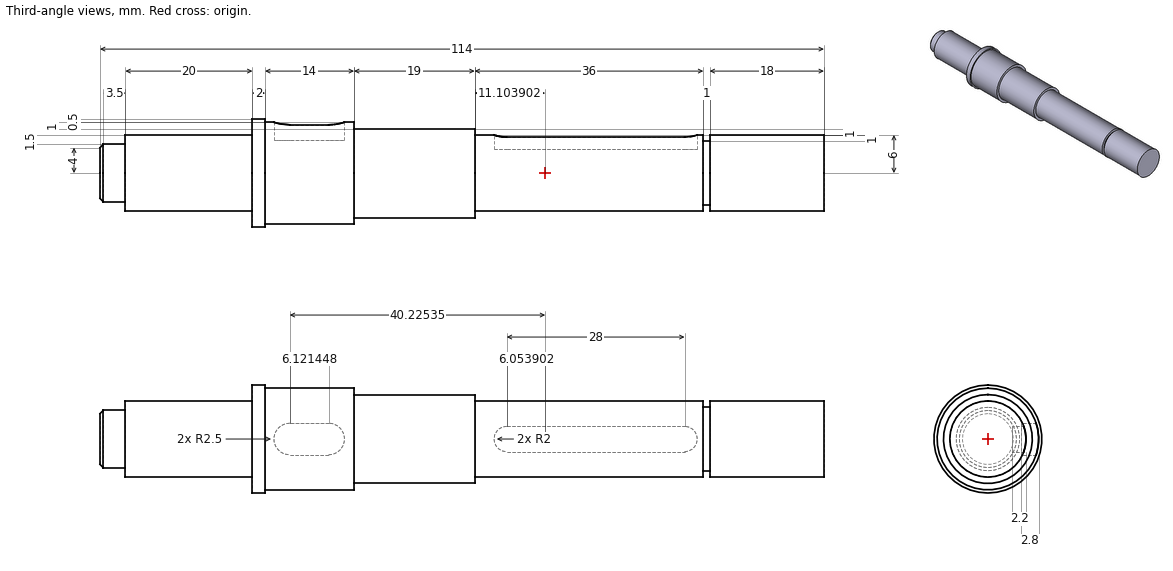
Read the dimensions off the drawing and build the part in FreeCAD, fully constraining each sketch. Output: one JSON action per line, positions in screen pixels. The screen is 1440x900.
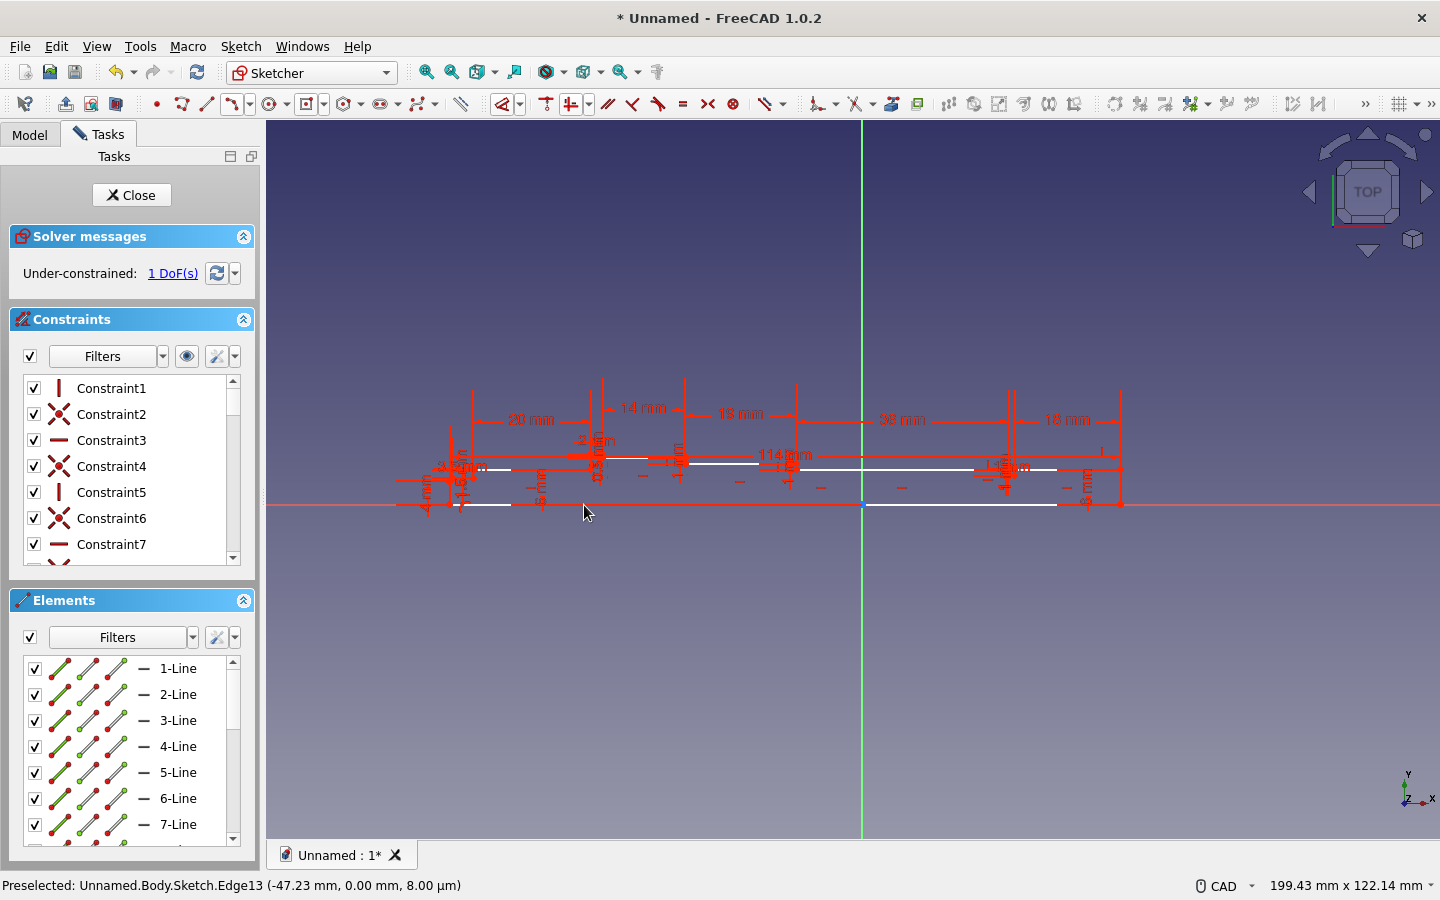
{"action": "scroll", "coordinate": [797, 470], "scroll_direction": "up", "scroll_amount": 4}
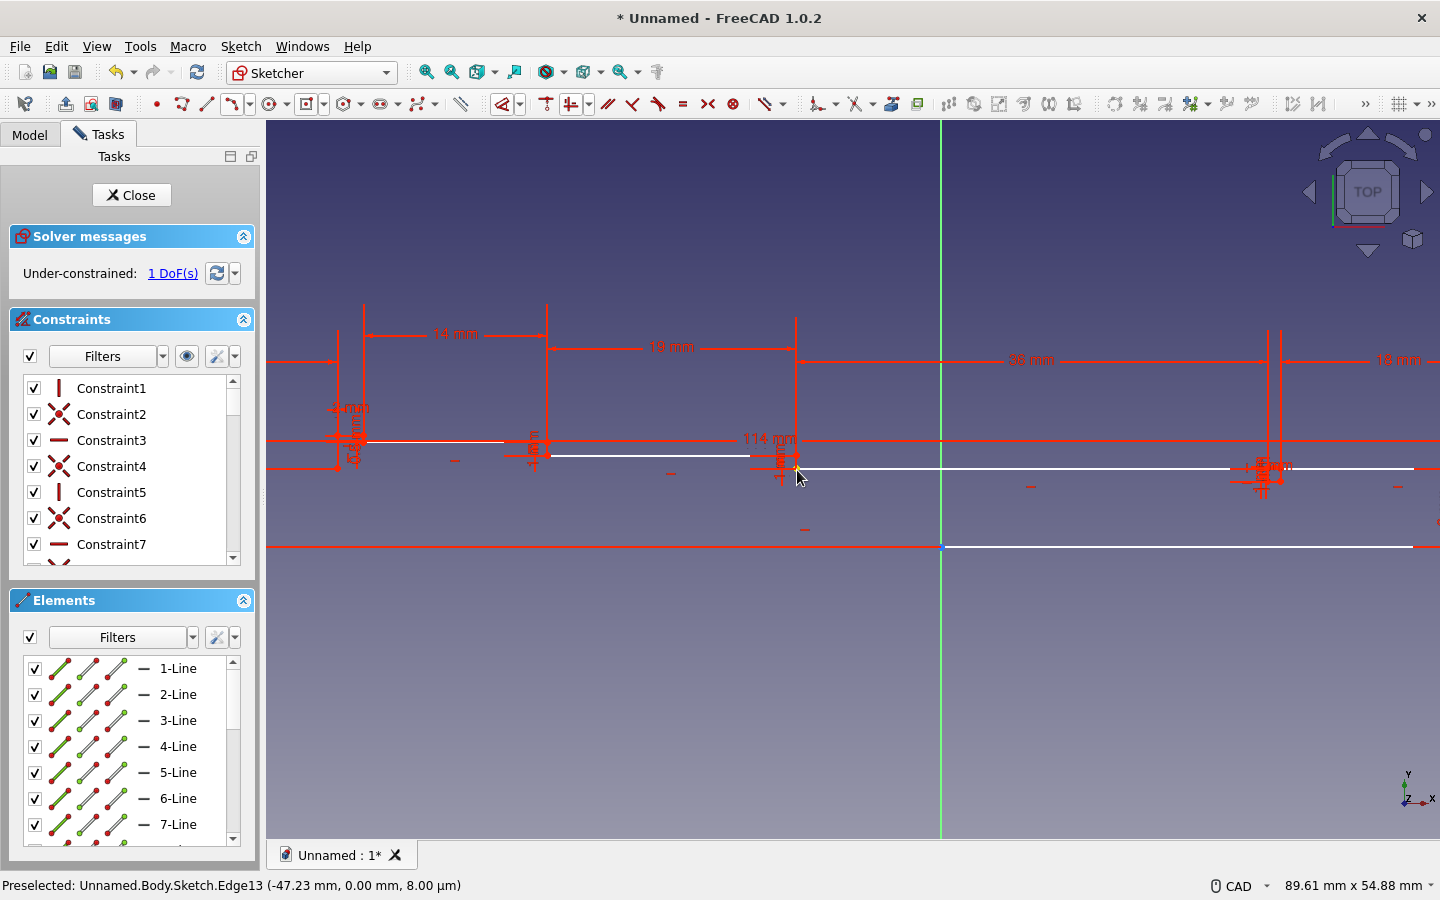
{"action": "left_click", "coordinate": [796, 469]}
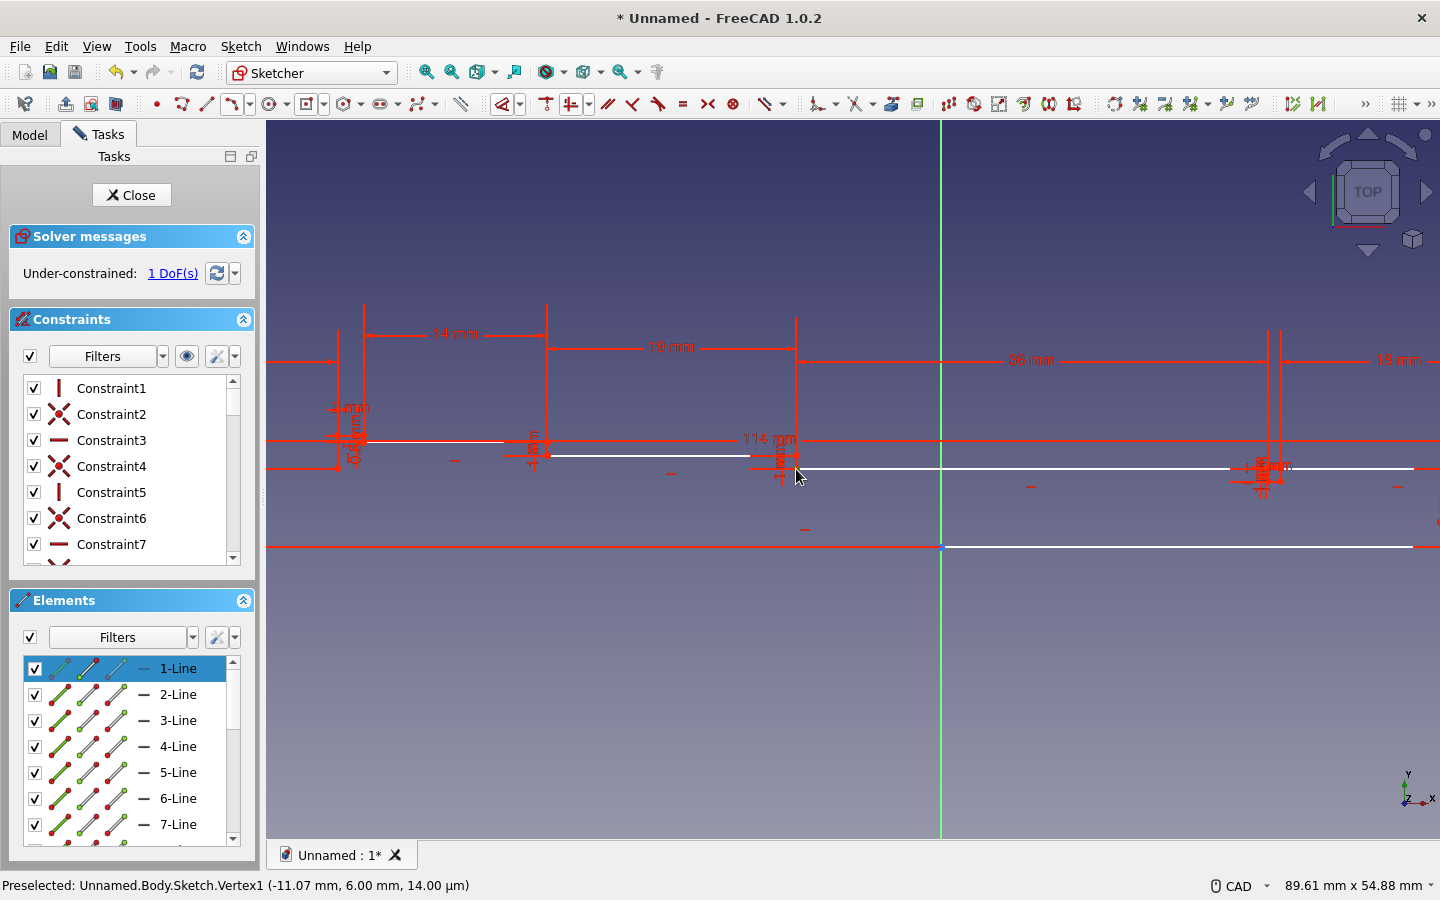
{"action": "key", "text": "l"}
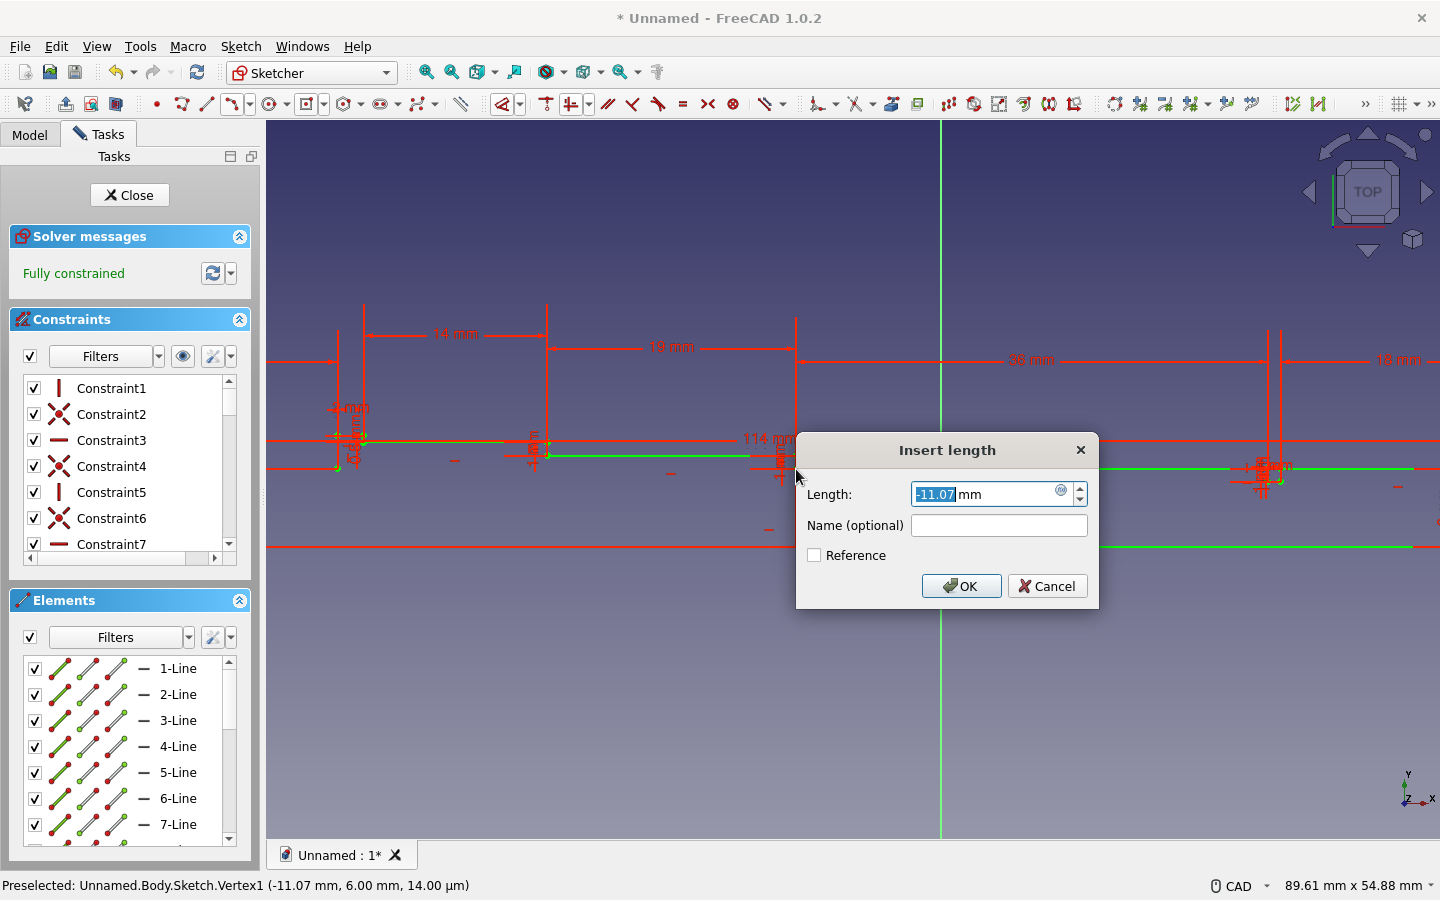
{"action": "type", "text": "-11.103902"}
{"action": "key", "text": "Return"}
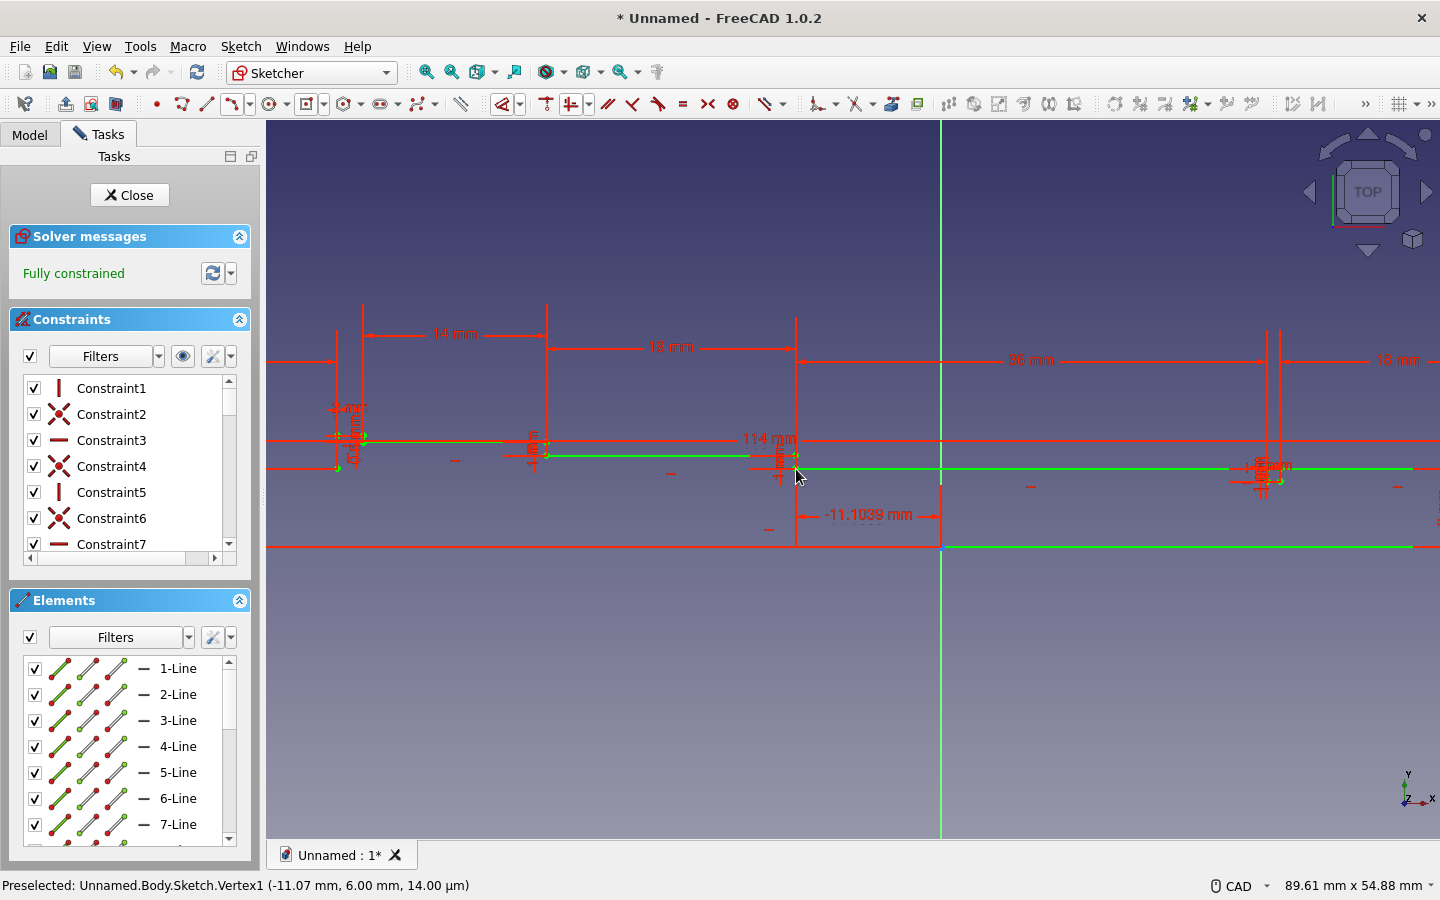
{"action": "left_click", "coordinate": [130, 195]}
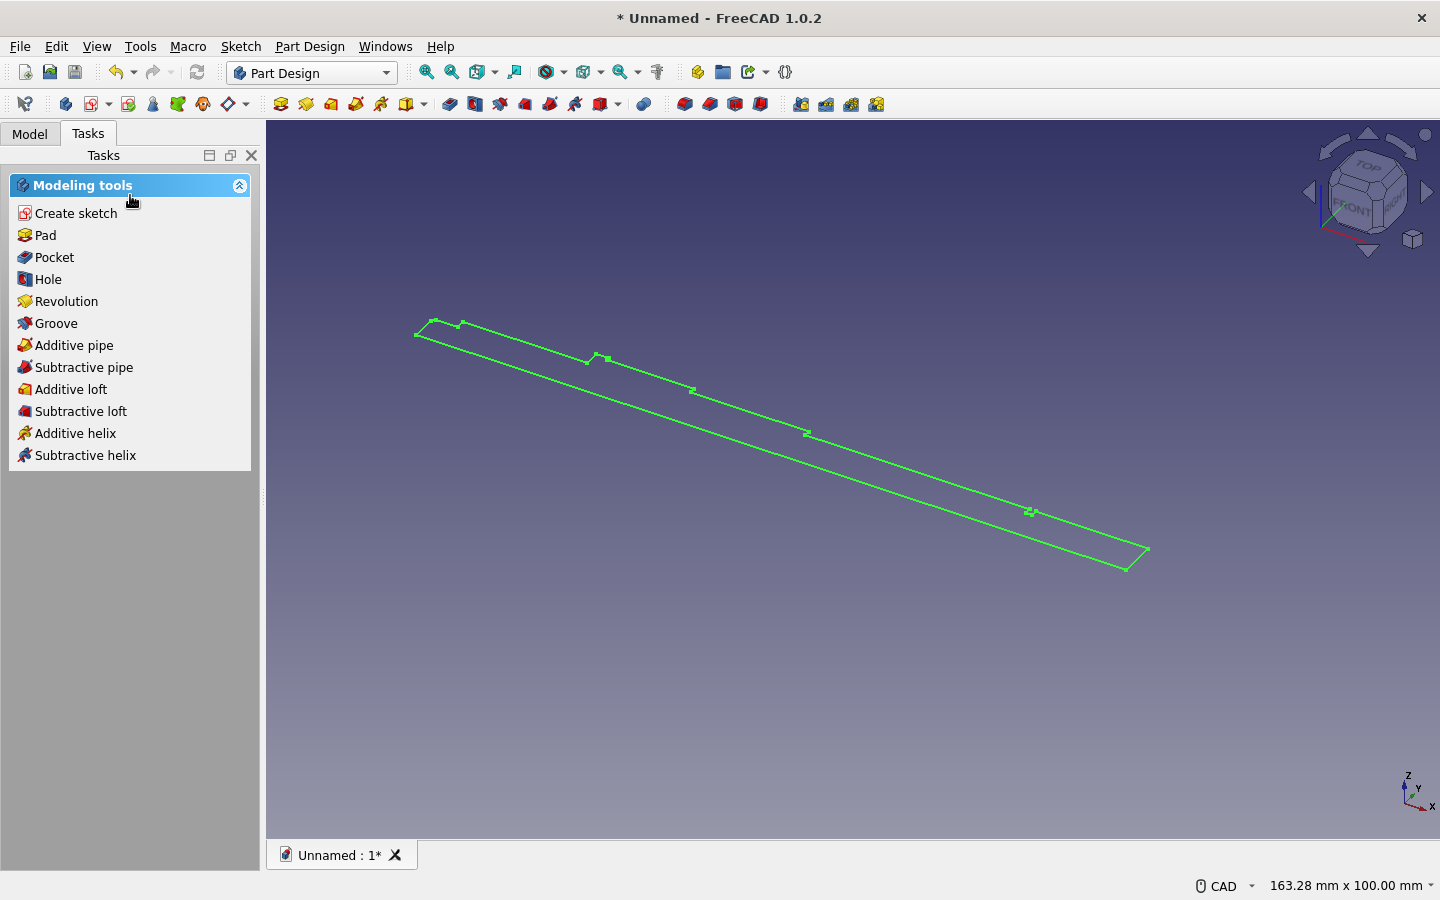
{"action": "left_click", "coordinate": [306, 104]}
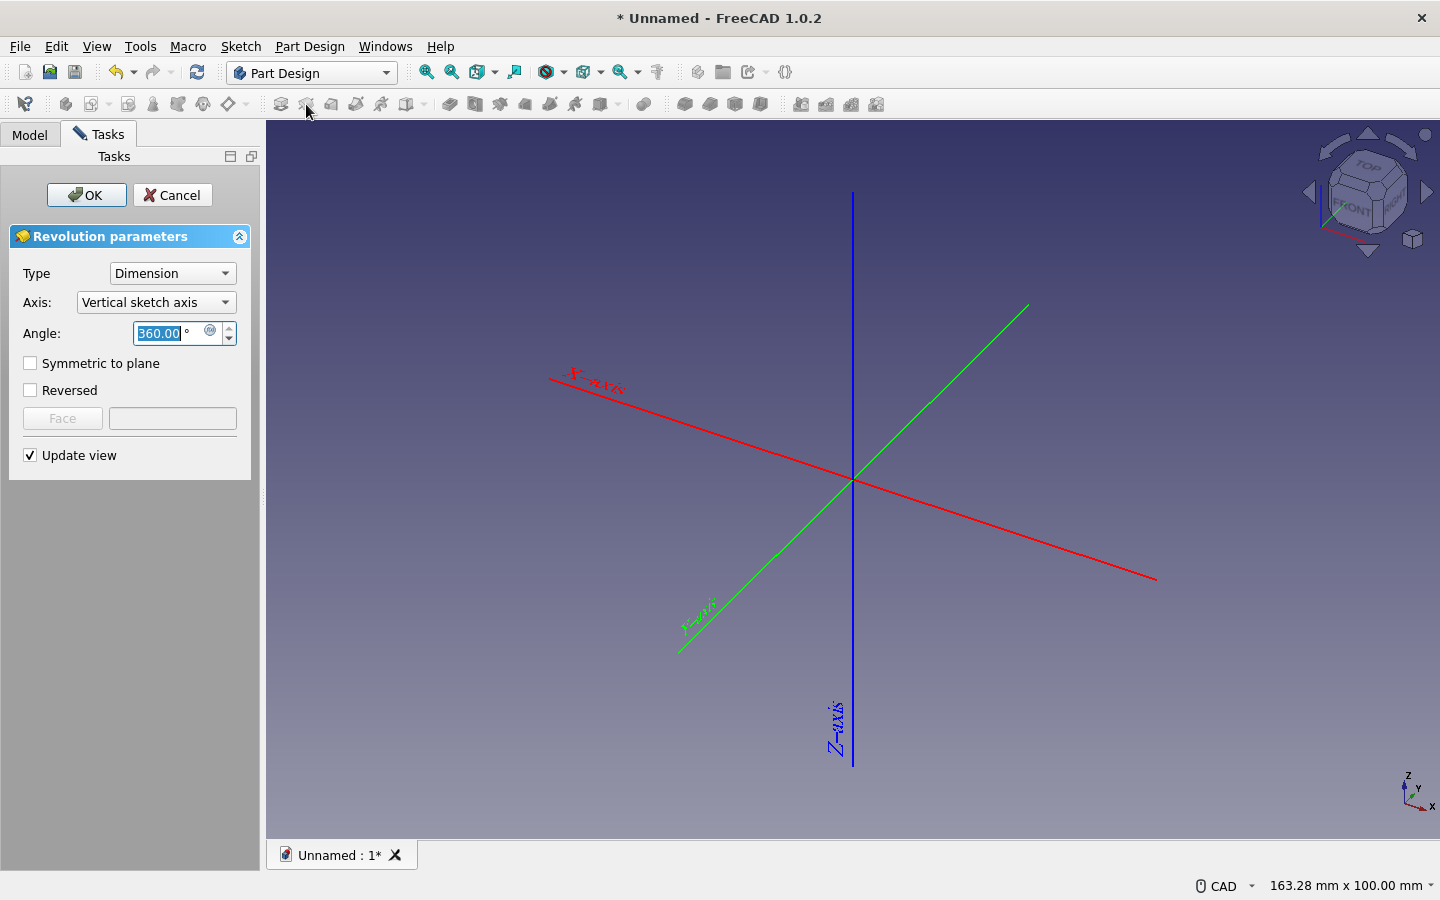
{"action": "left_click", "coordinate": [157, 302]}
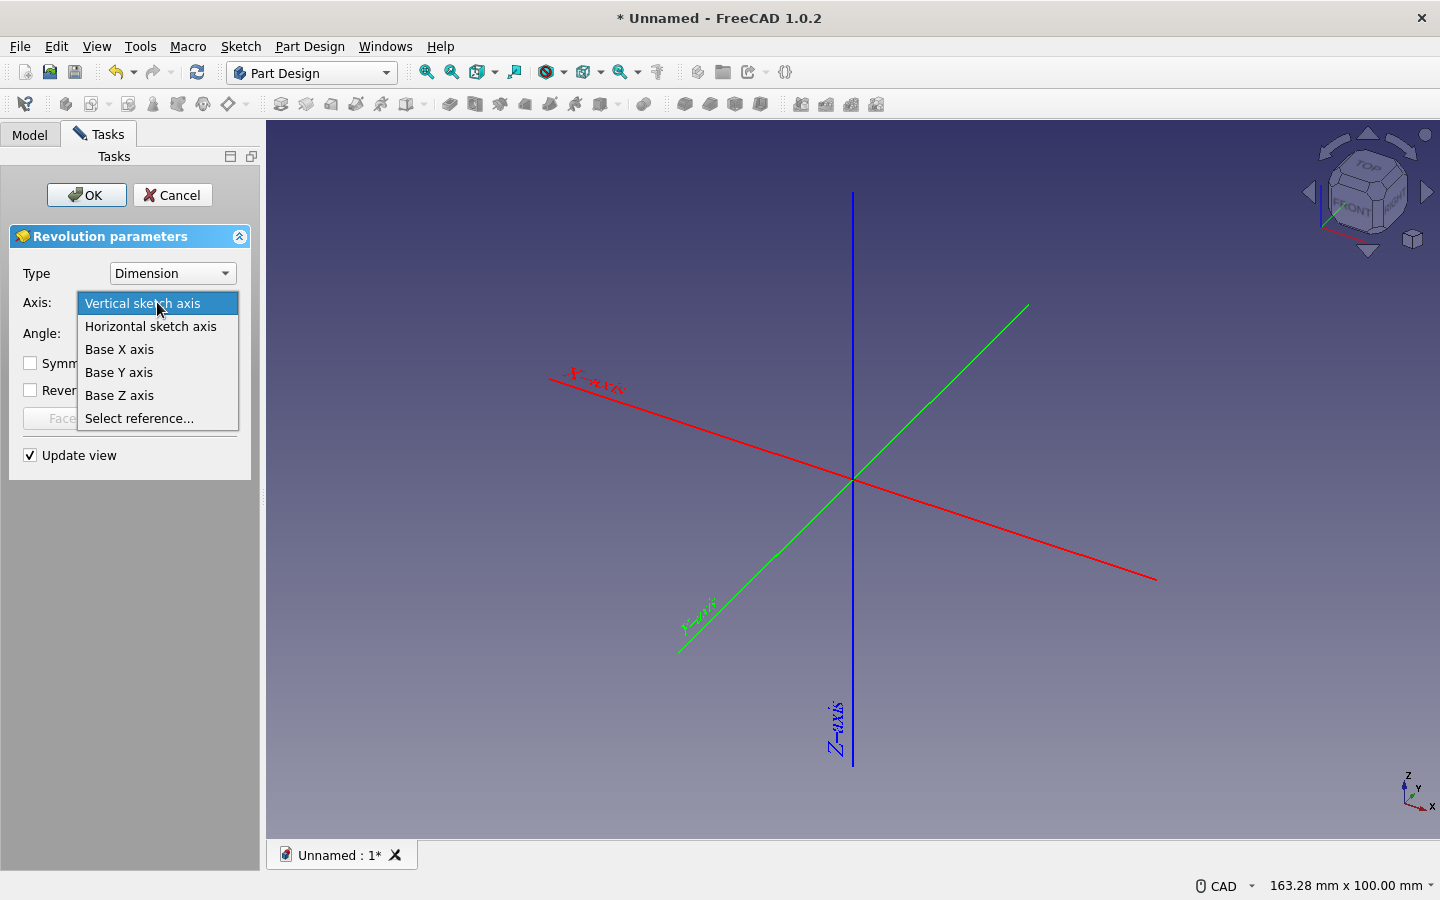
{"action": "left_click", "coordinate": [156, 326]}